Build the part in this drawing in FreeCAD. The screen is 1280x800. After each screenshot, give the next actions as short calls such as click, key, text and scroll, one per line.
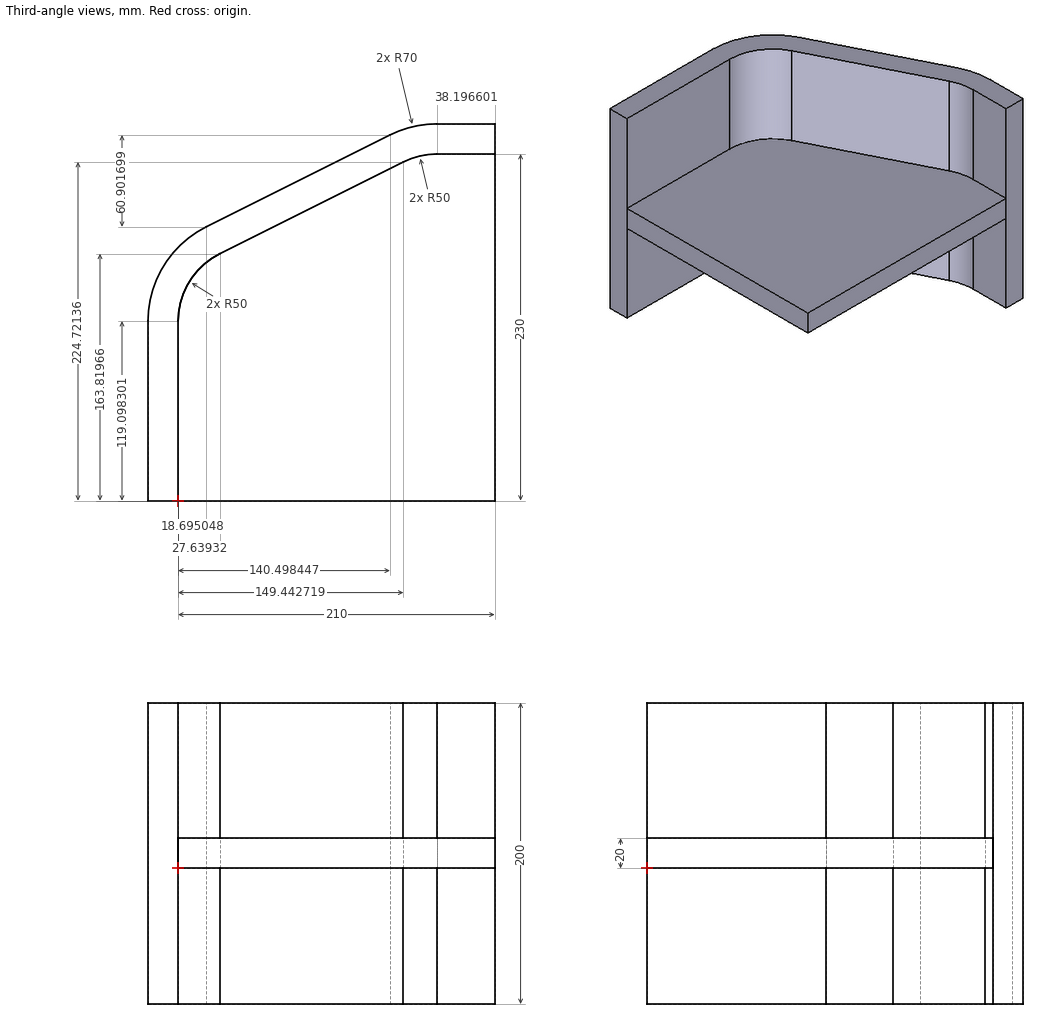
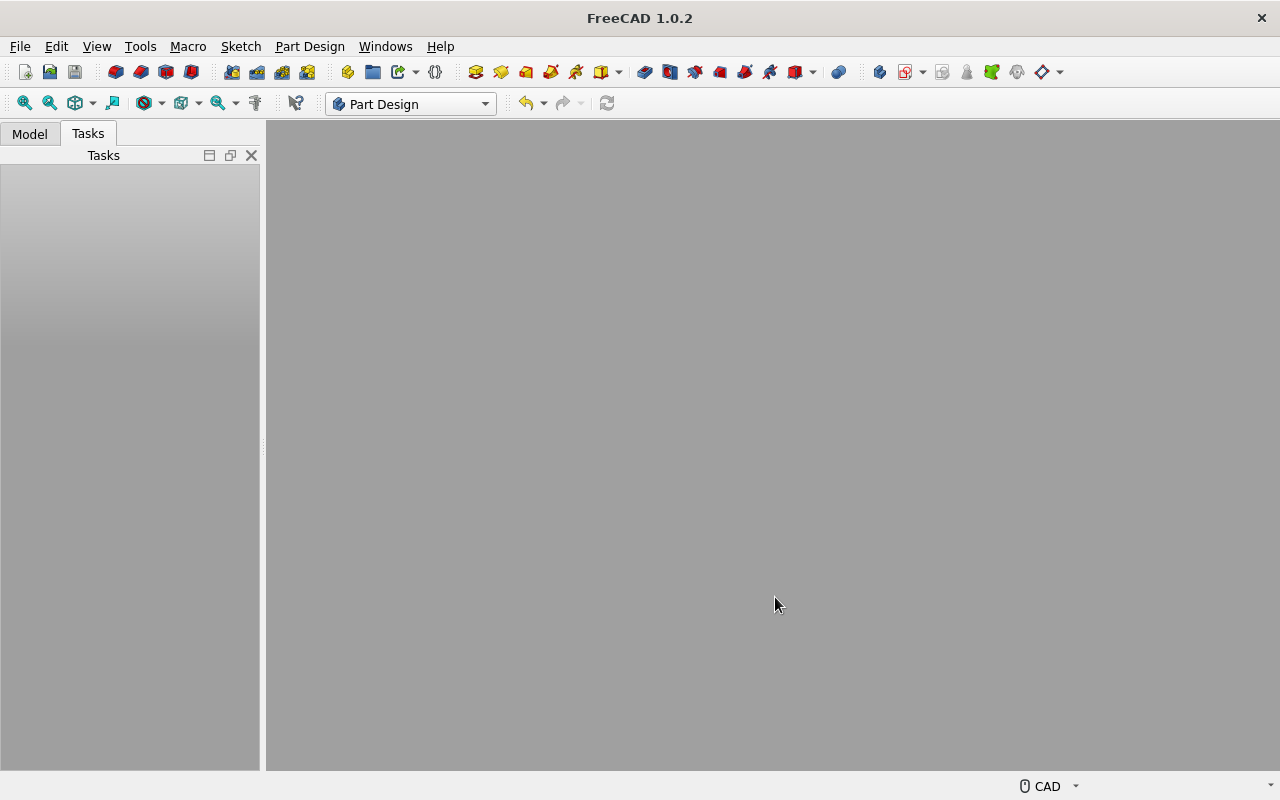
click(25, 72)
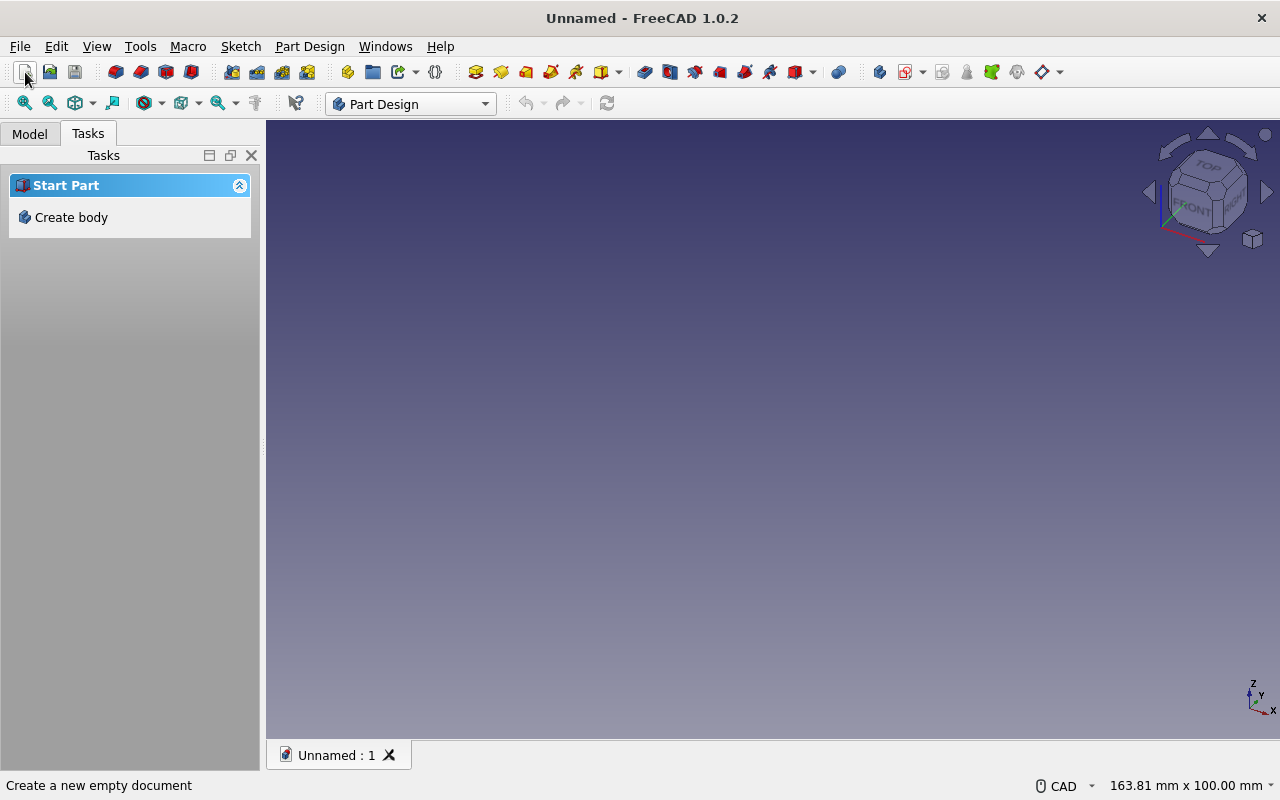
click(904, 72)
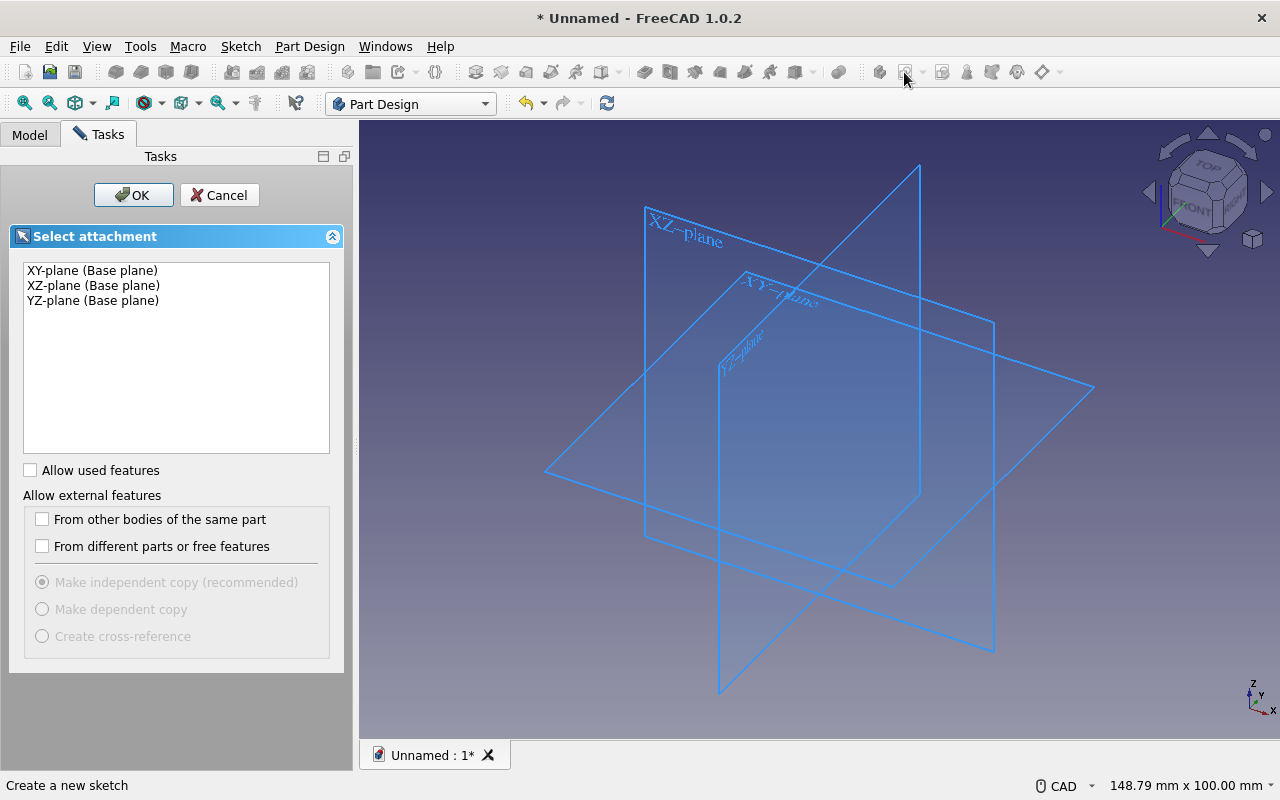
click(84, 270)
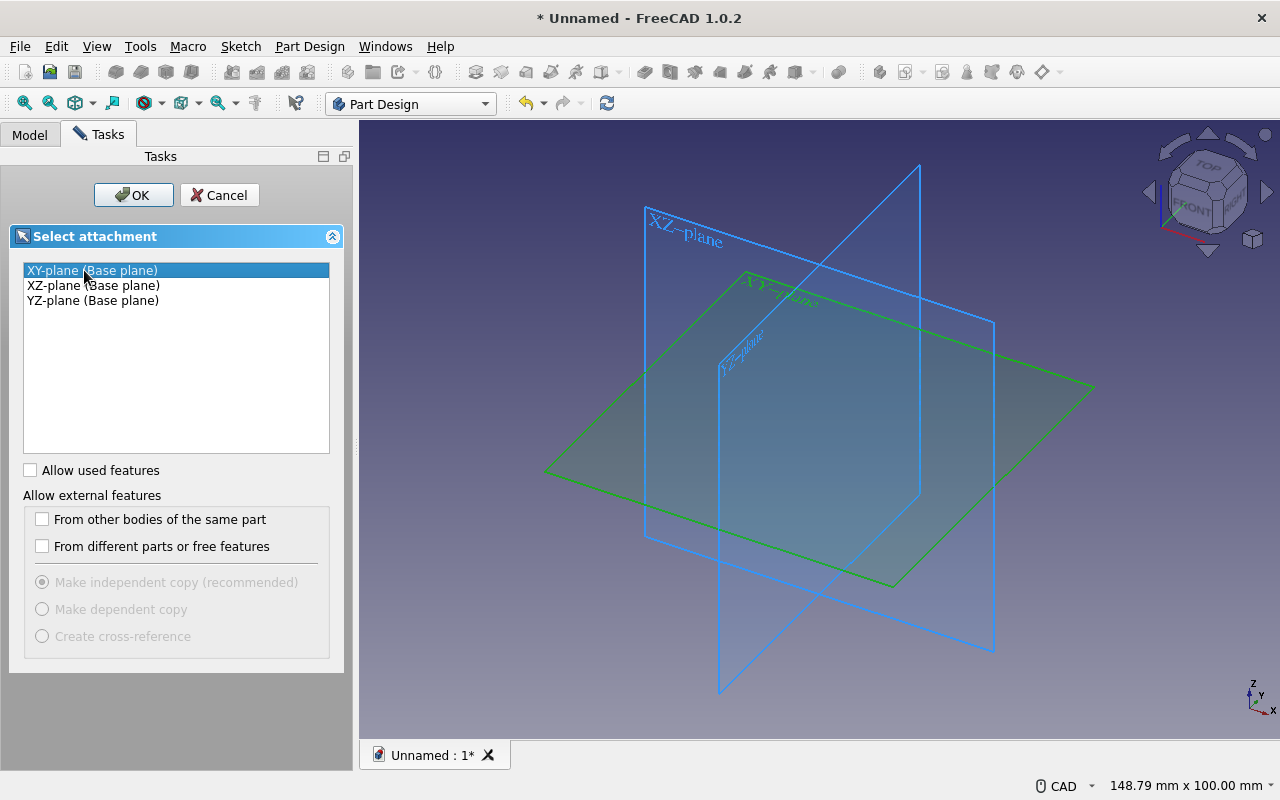
click(134, 195)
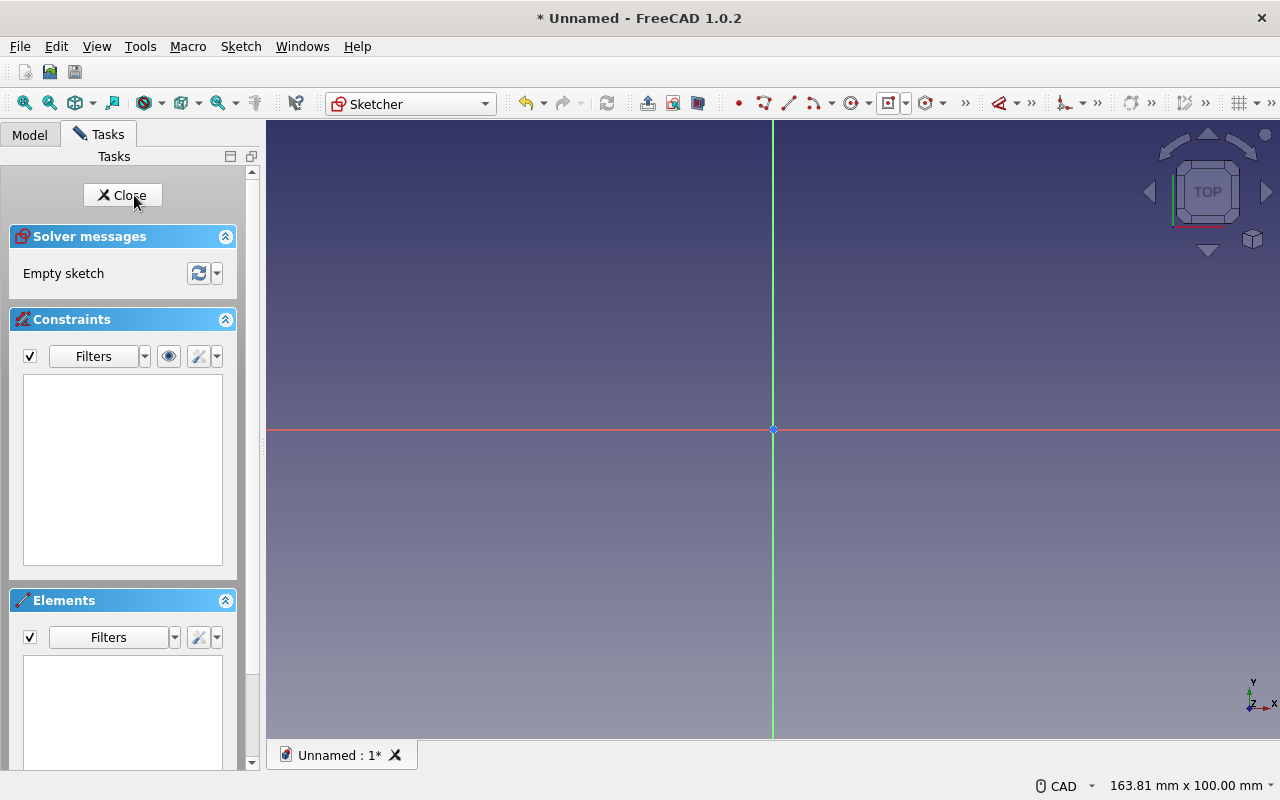
scroll(395, 711, down, 6)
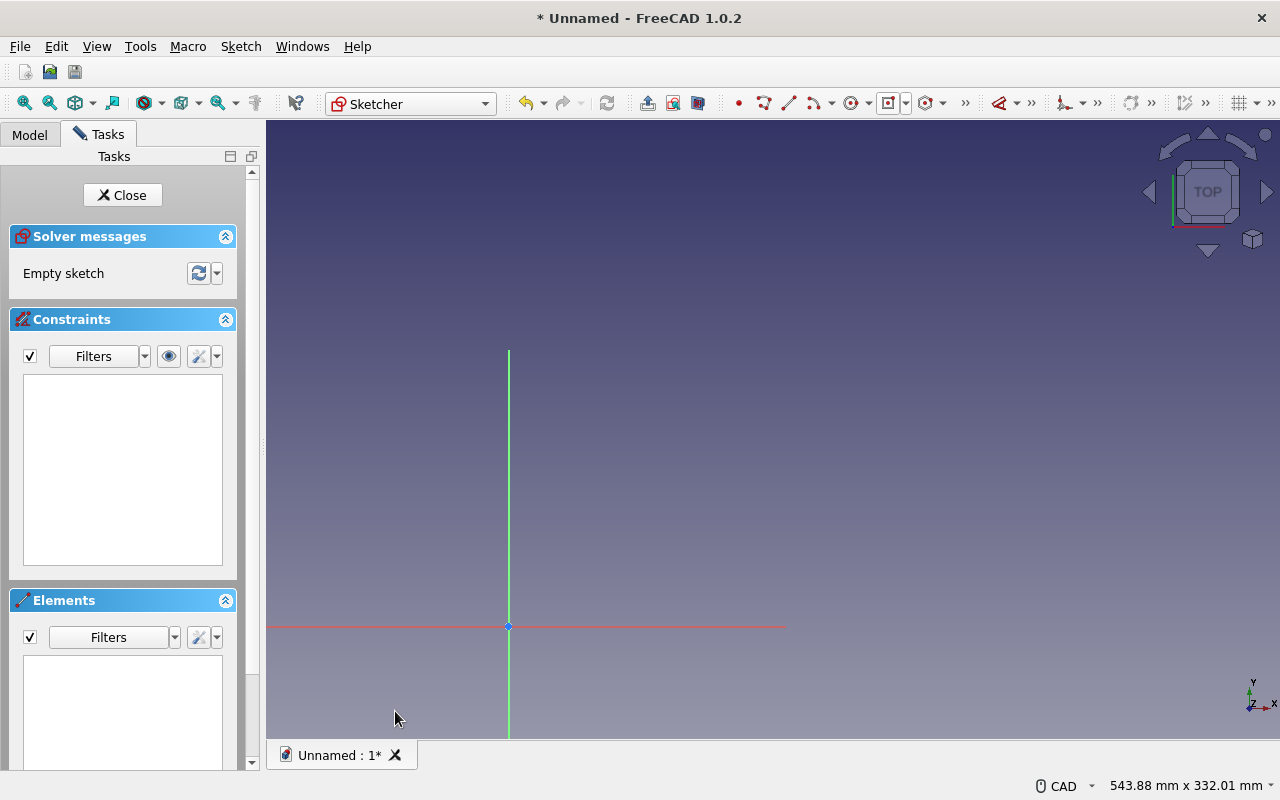
click(789, 104)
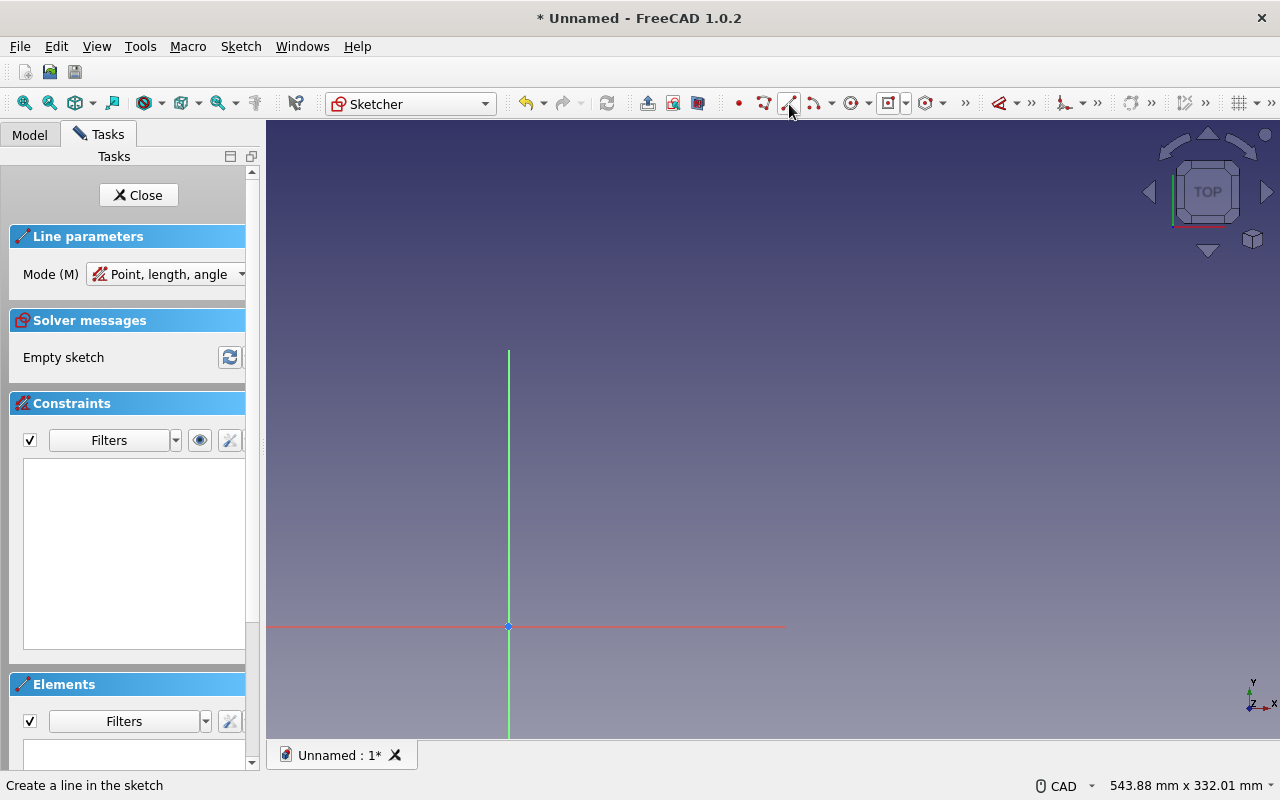
click(788, 208)
click(560, 321)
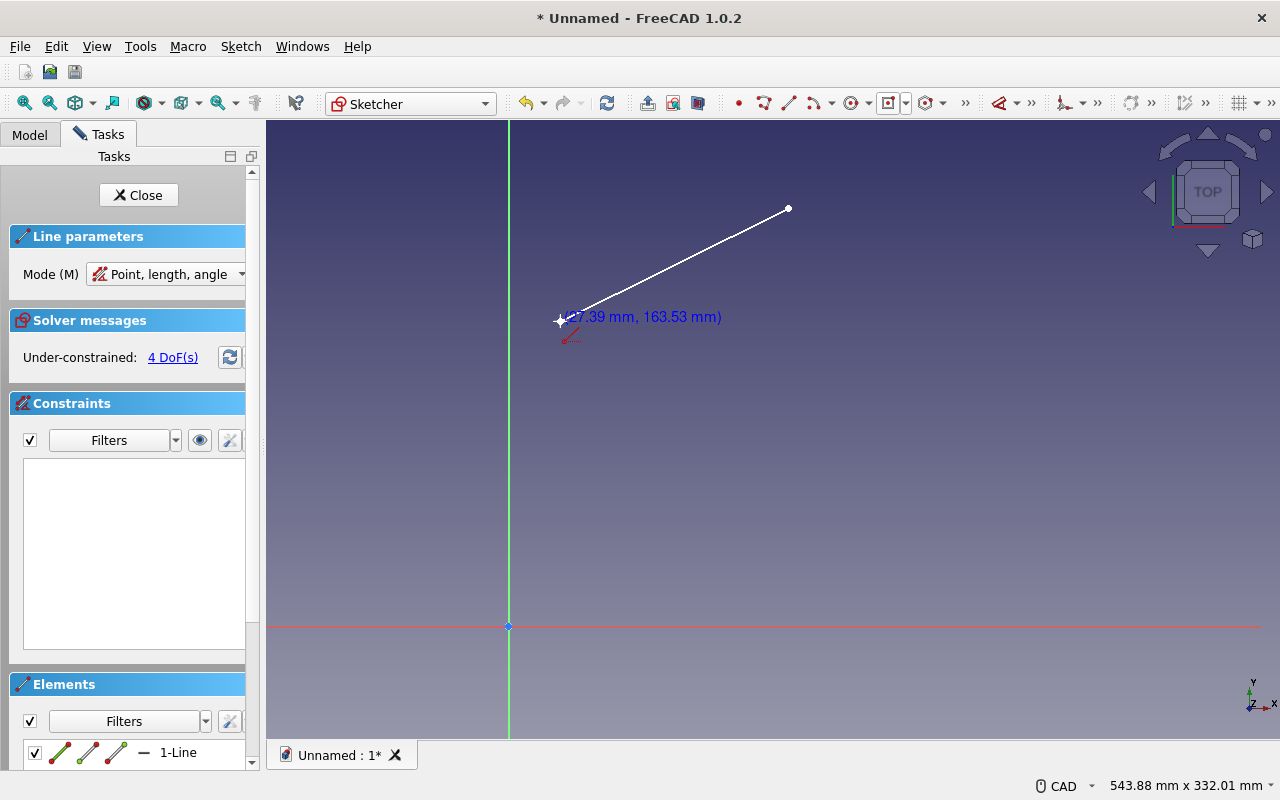
click(764, 104)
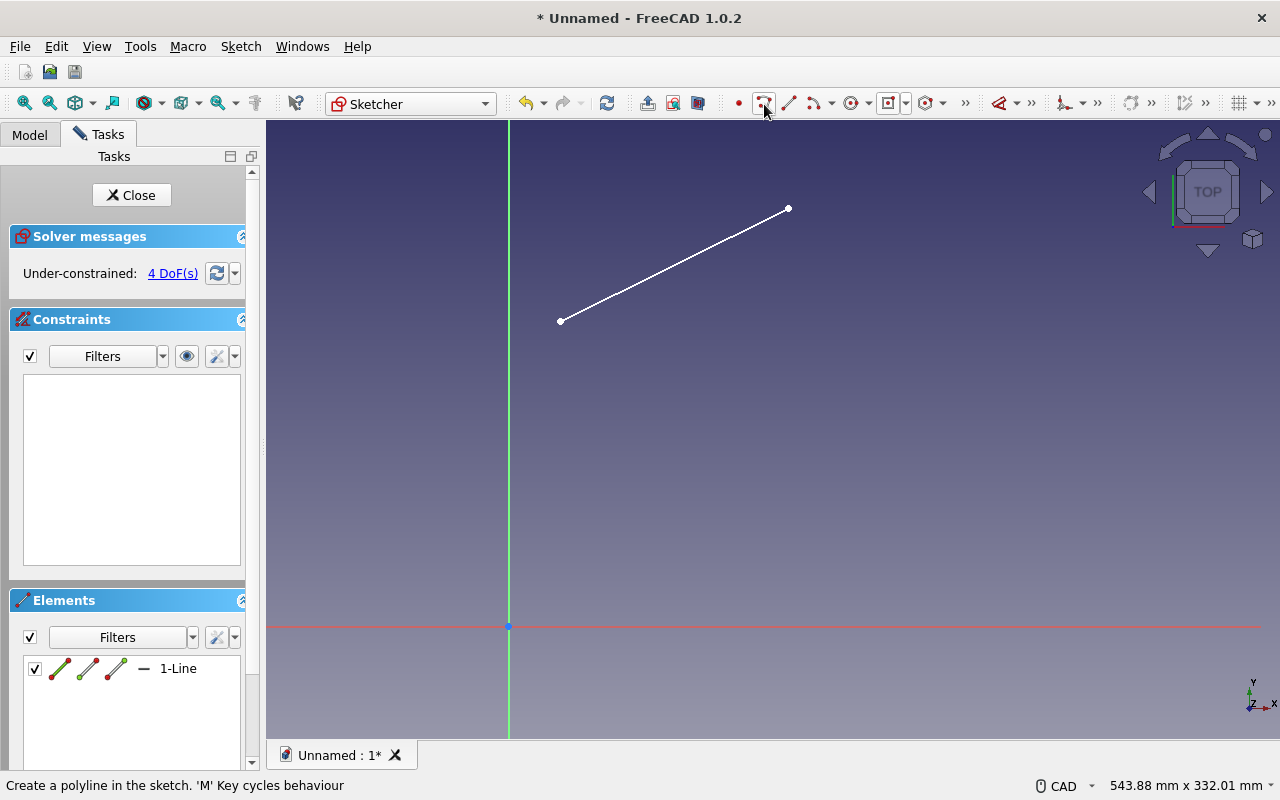
click(509, 405)
click(509, 627)
click(900, 618)
click(900, 198)
click(829, 198)
right_click(829, 198)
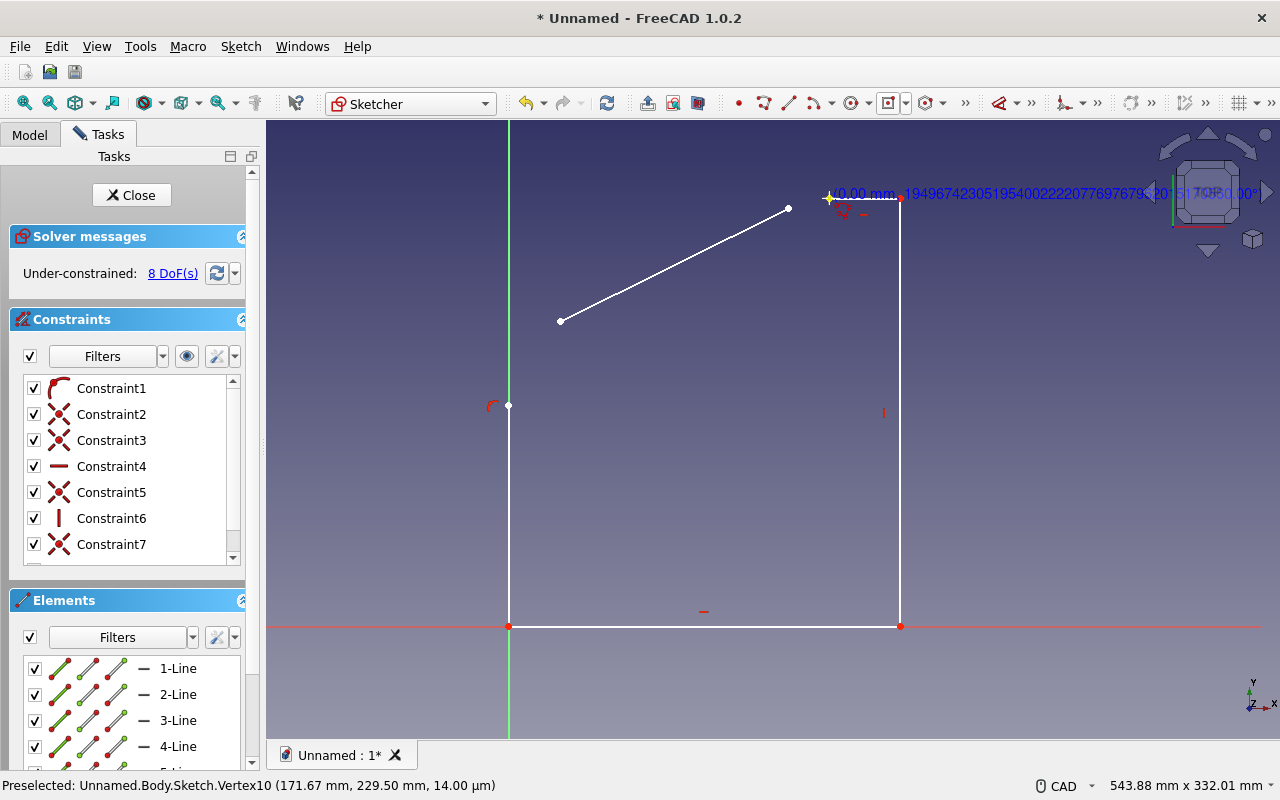
click(832, 104)